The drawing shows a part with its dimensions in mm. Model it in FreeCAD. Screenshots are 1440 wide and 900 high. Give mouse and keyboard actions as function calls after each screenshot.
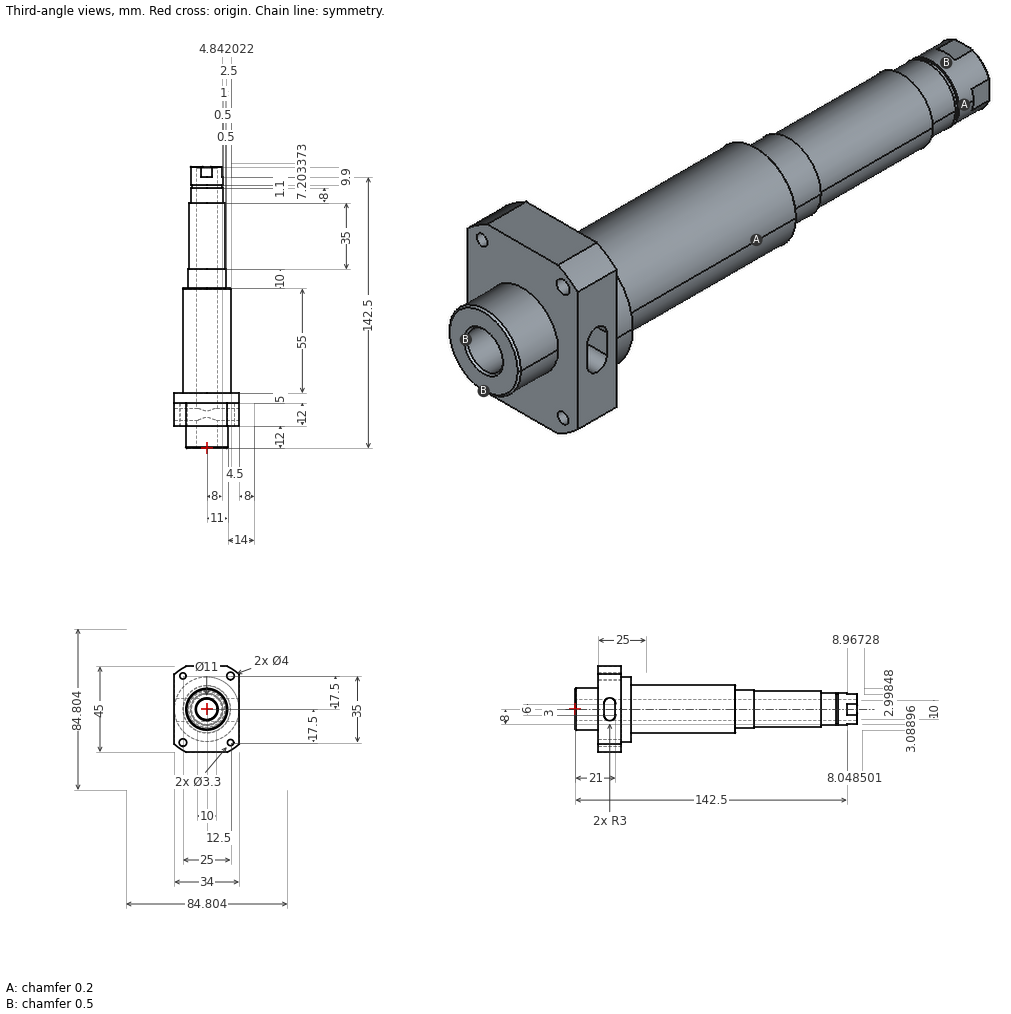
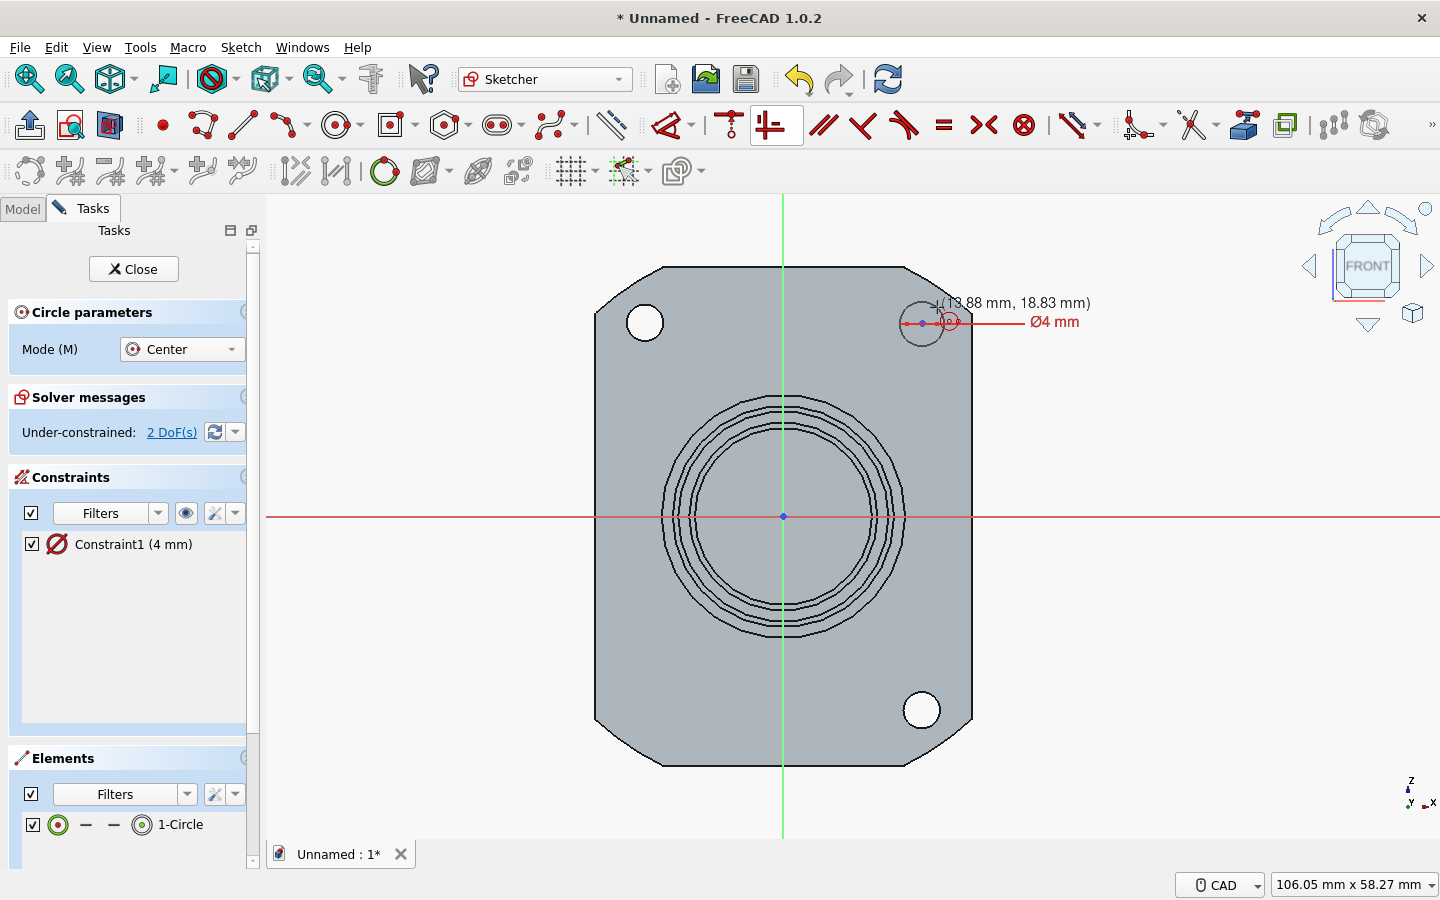
click(645, 710)
move(661, 695)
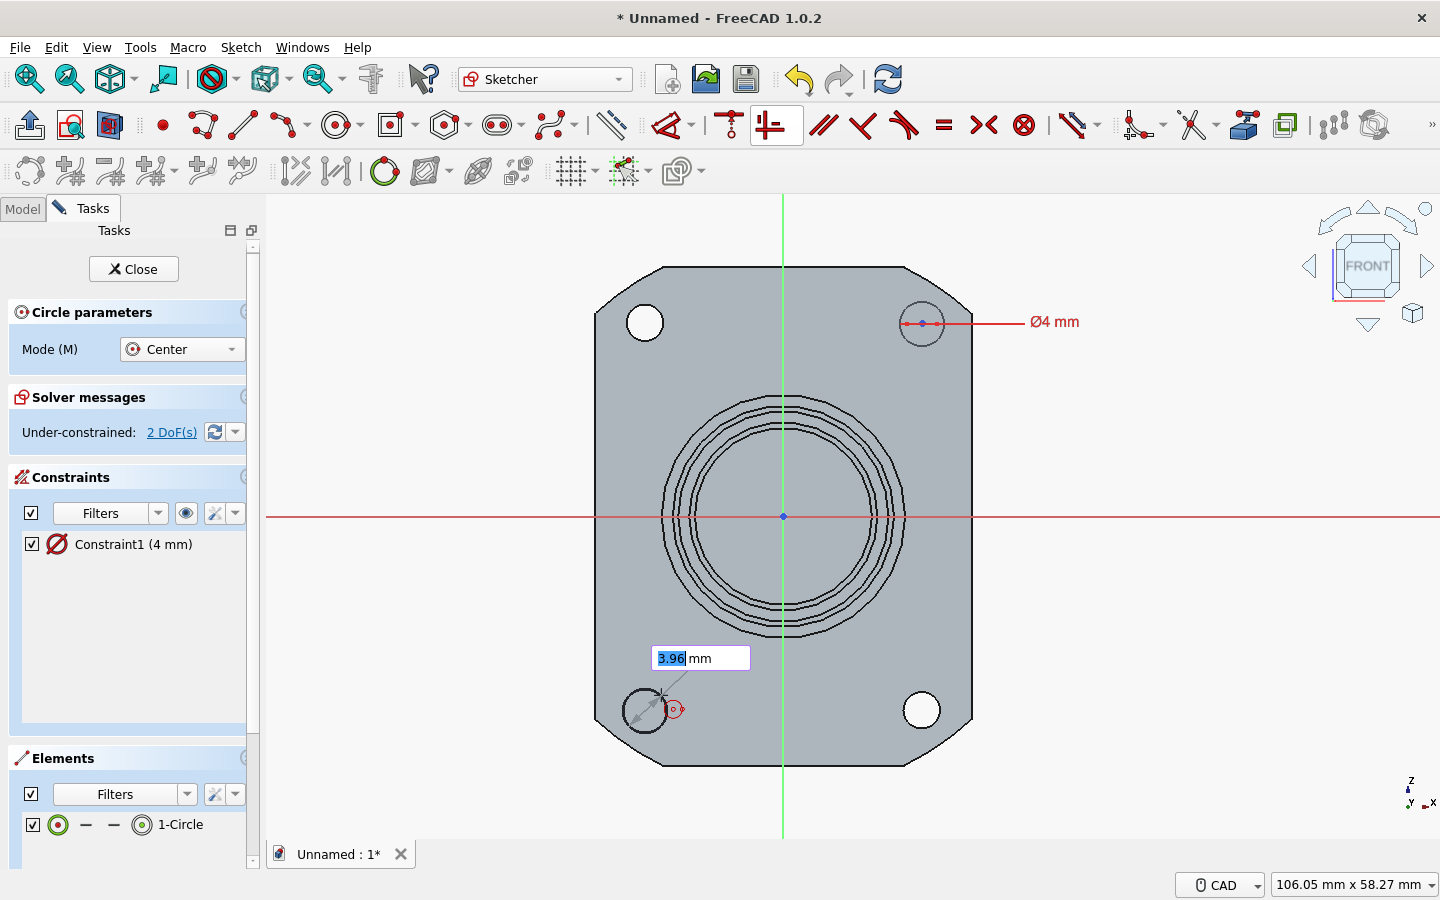
text(4)
key(Return)
key(Escape)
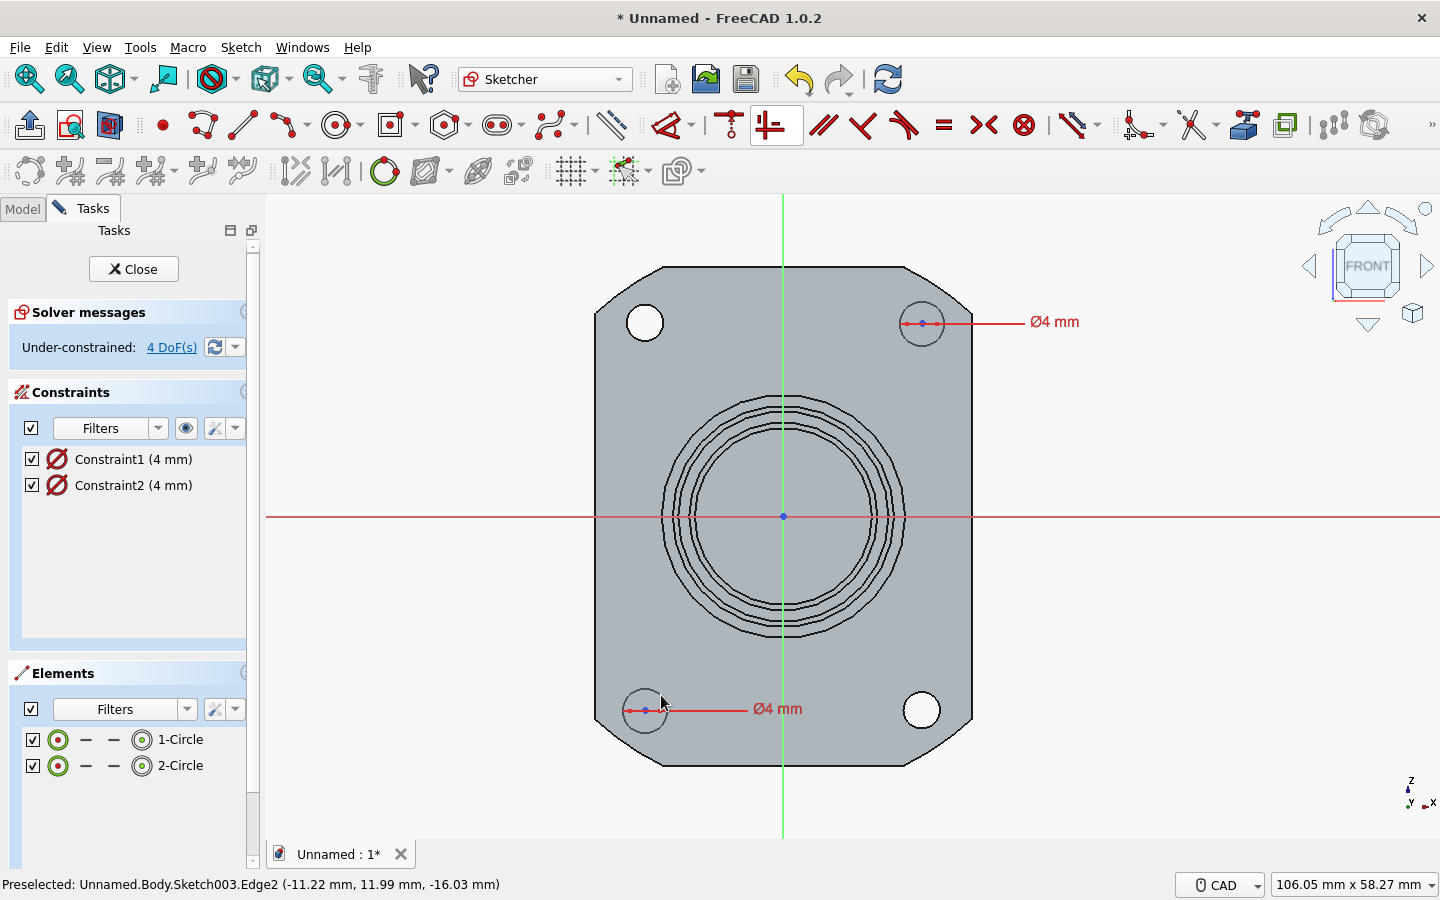
key(d)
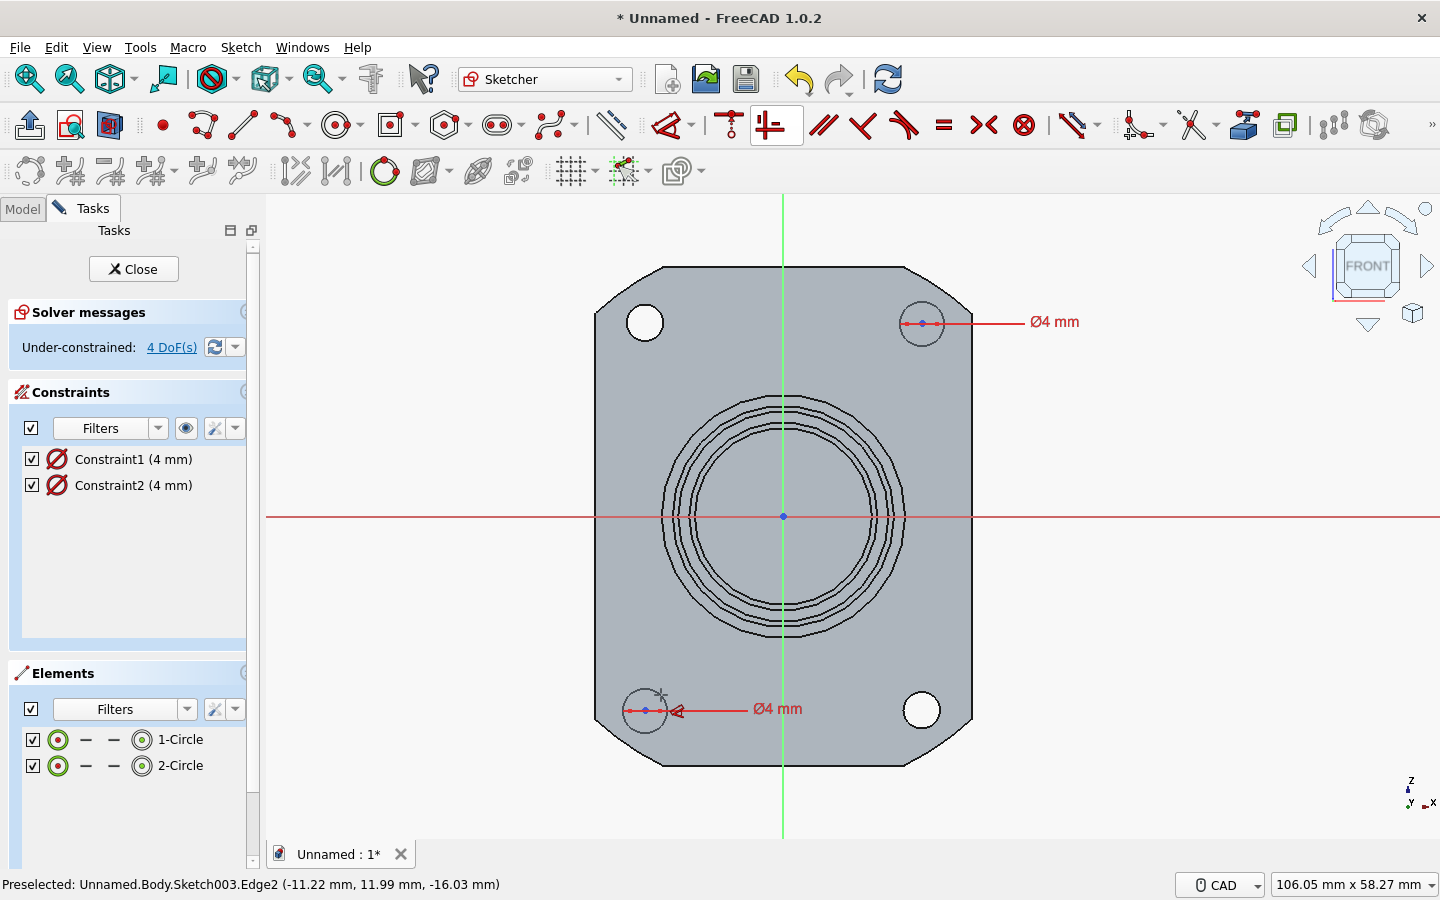
click(922, 324)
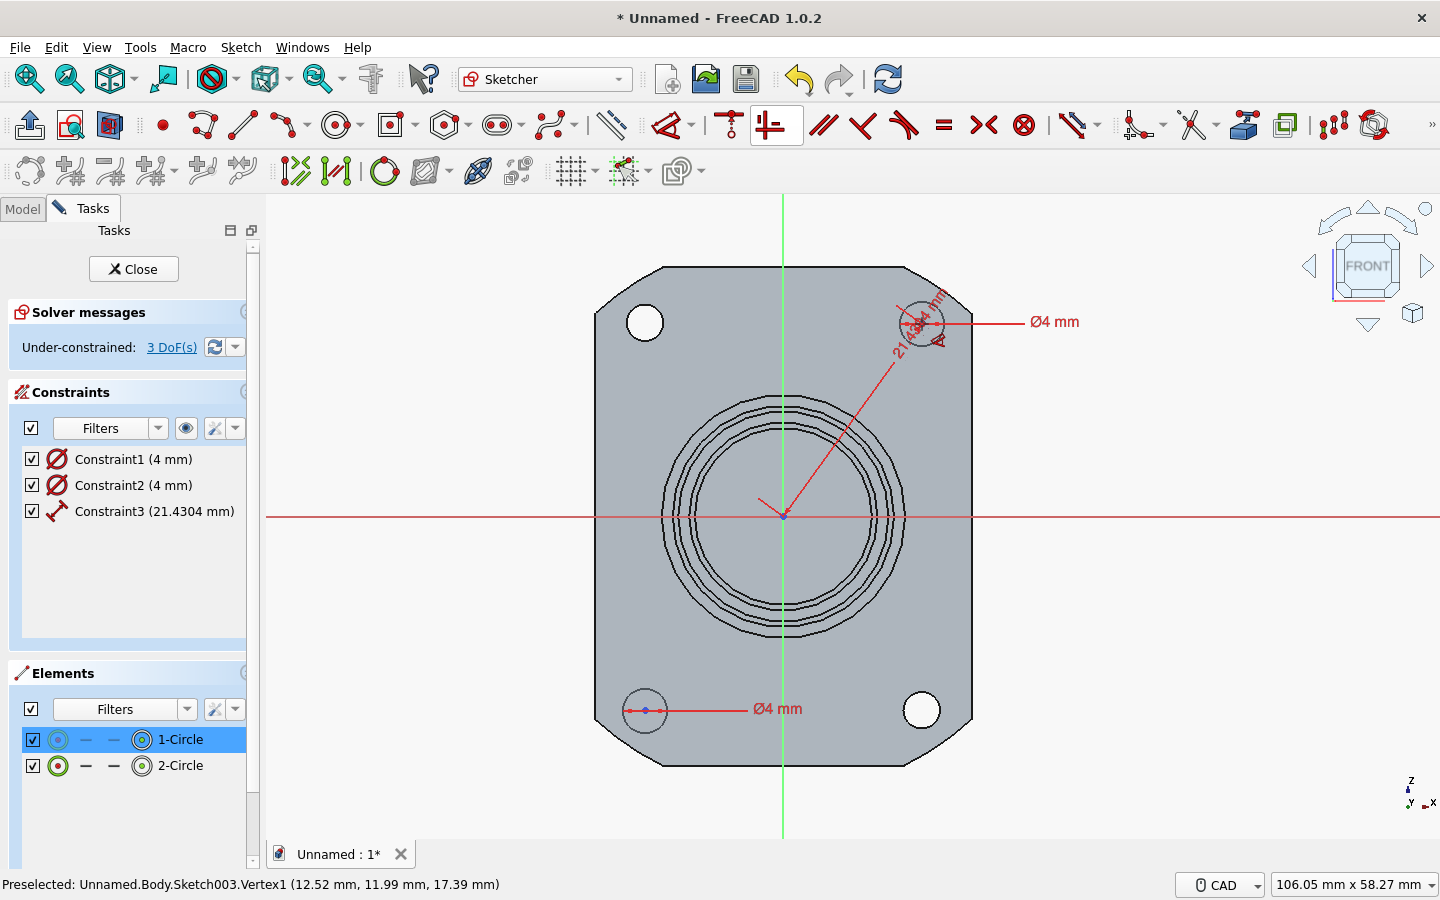
click(645, 711)
click(720, 745)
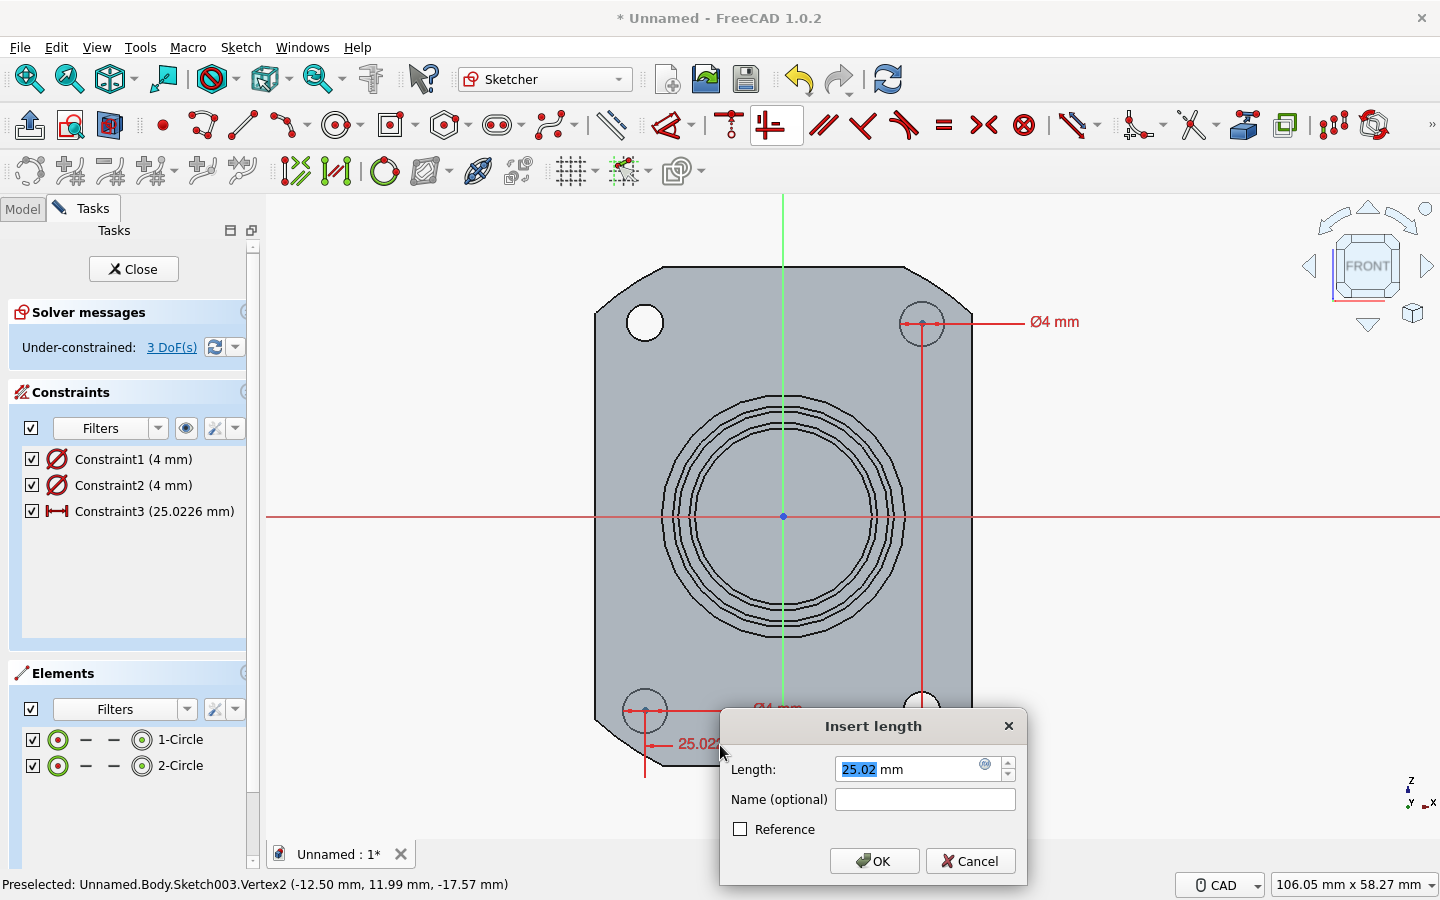
text(25)
key(Return)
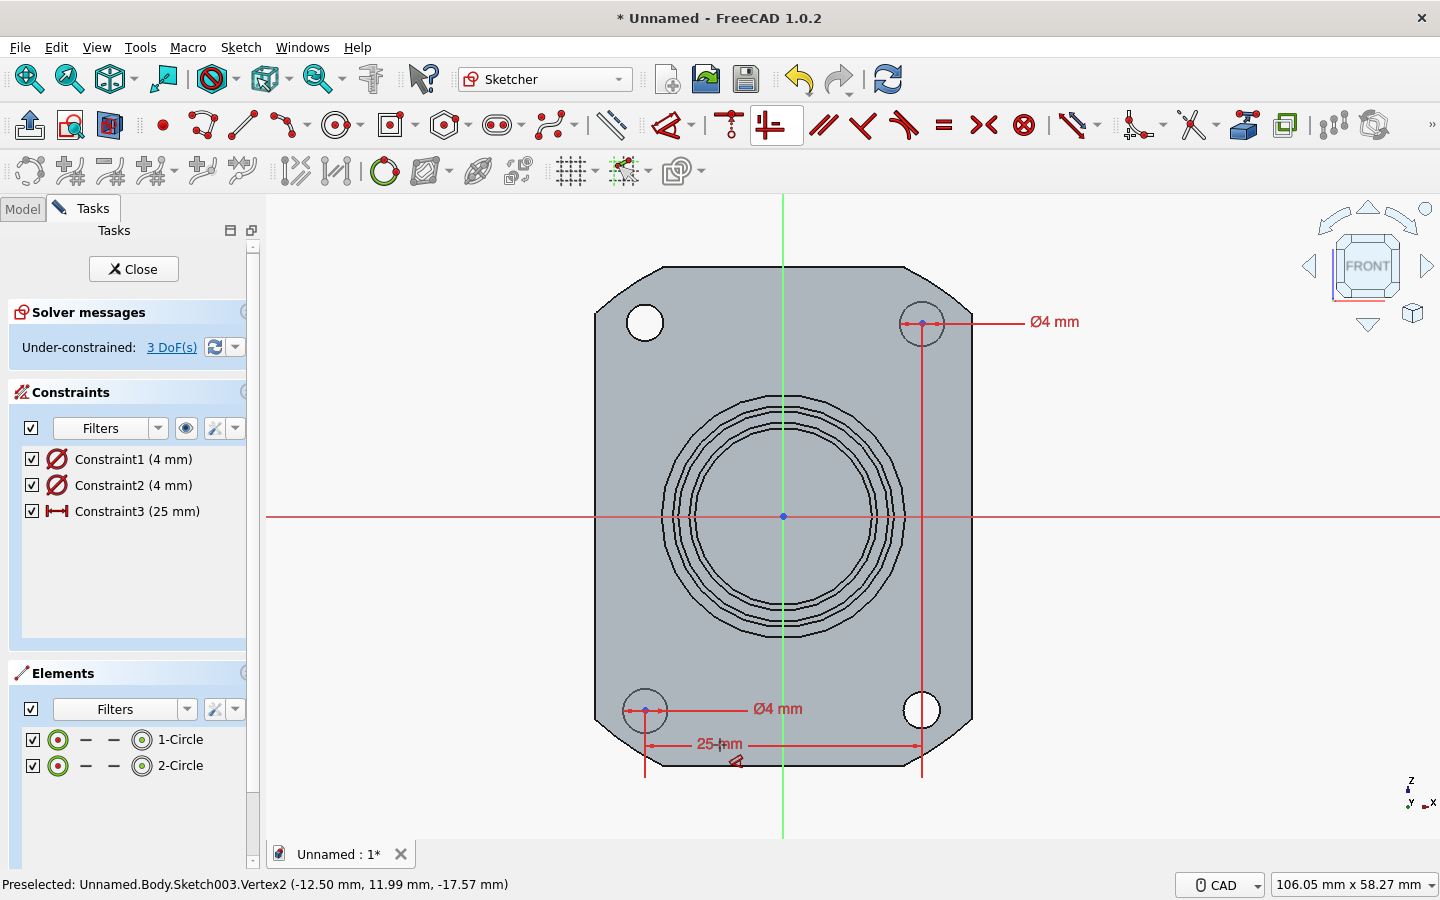
click(922, 324)